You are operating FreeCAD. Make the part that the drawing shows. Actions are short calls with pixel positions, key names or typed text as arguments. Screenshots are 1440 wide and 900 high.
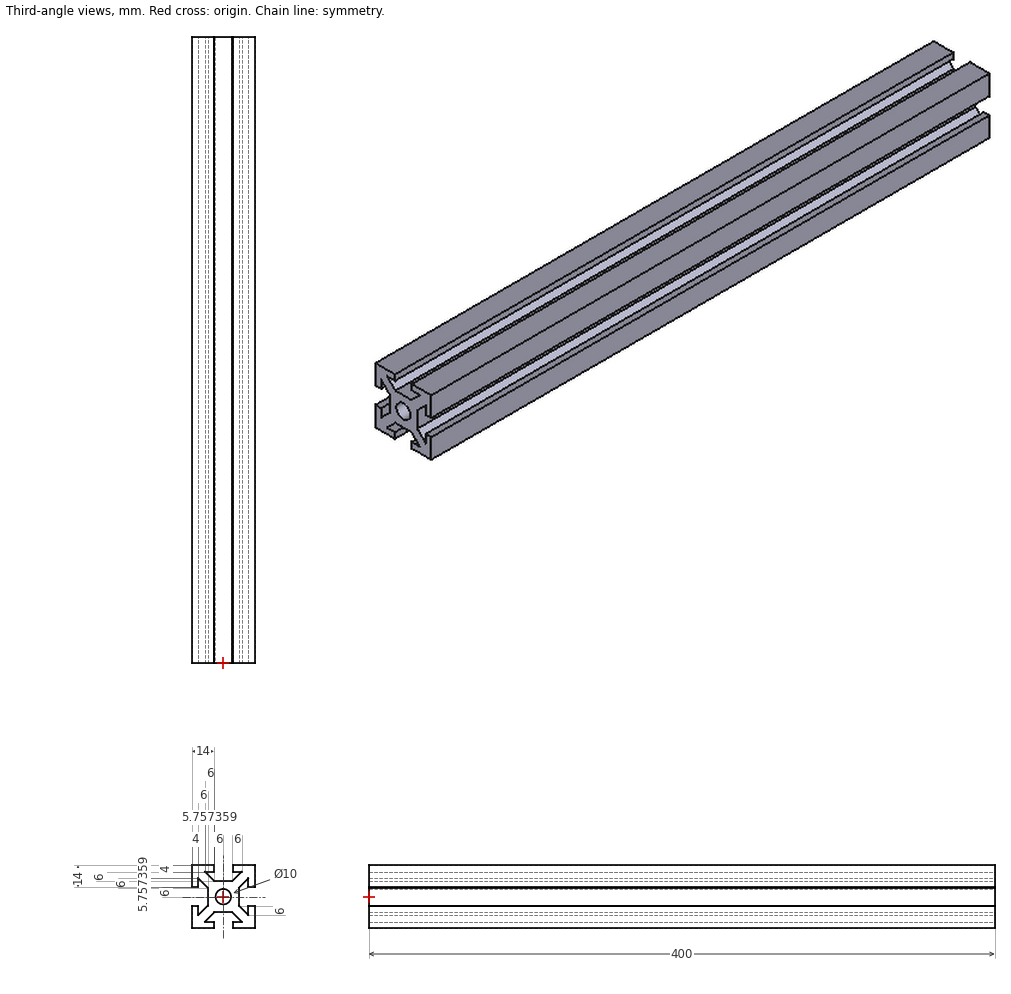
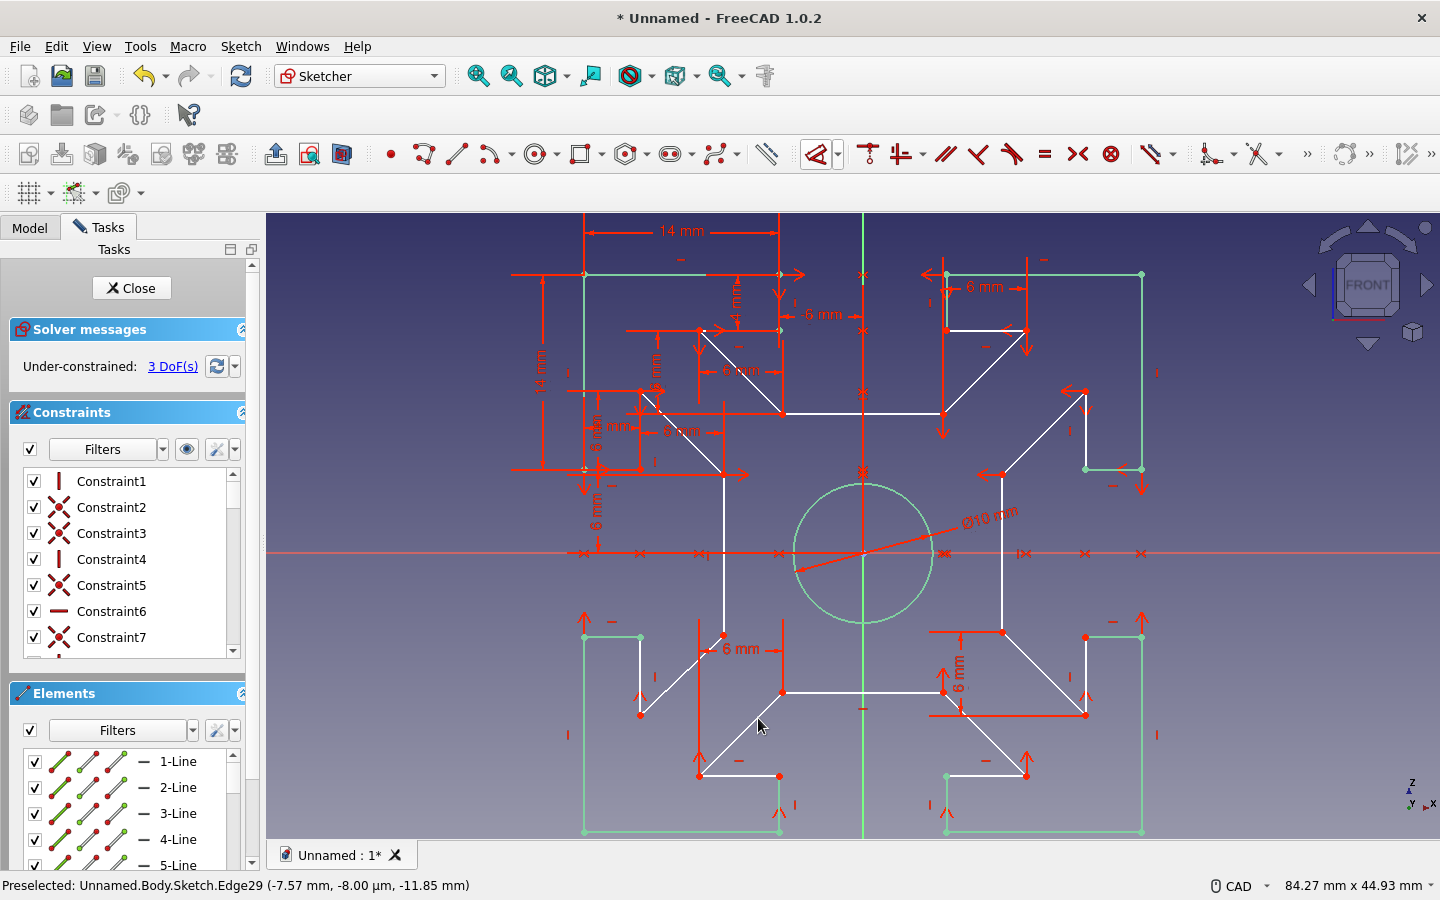
click(665, 692)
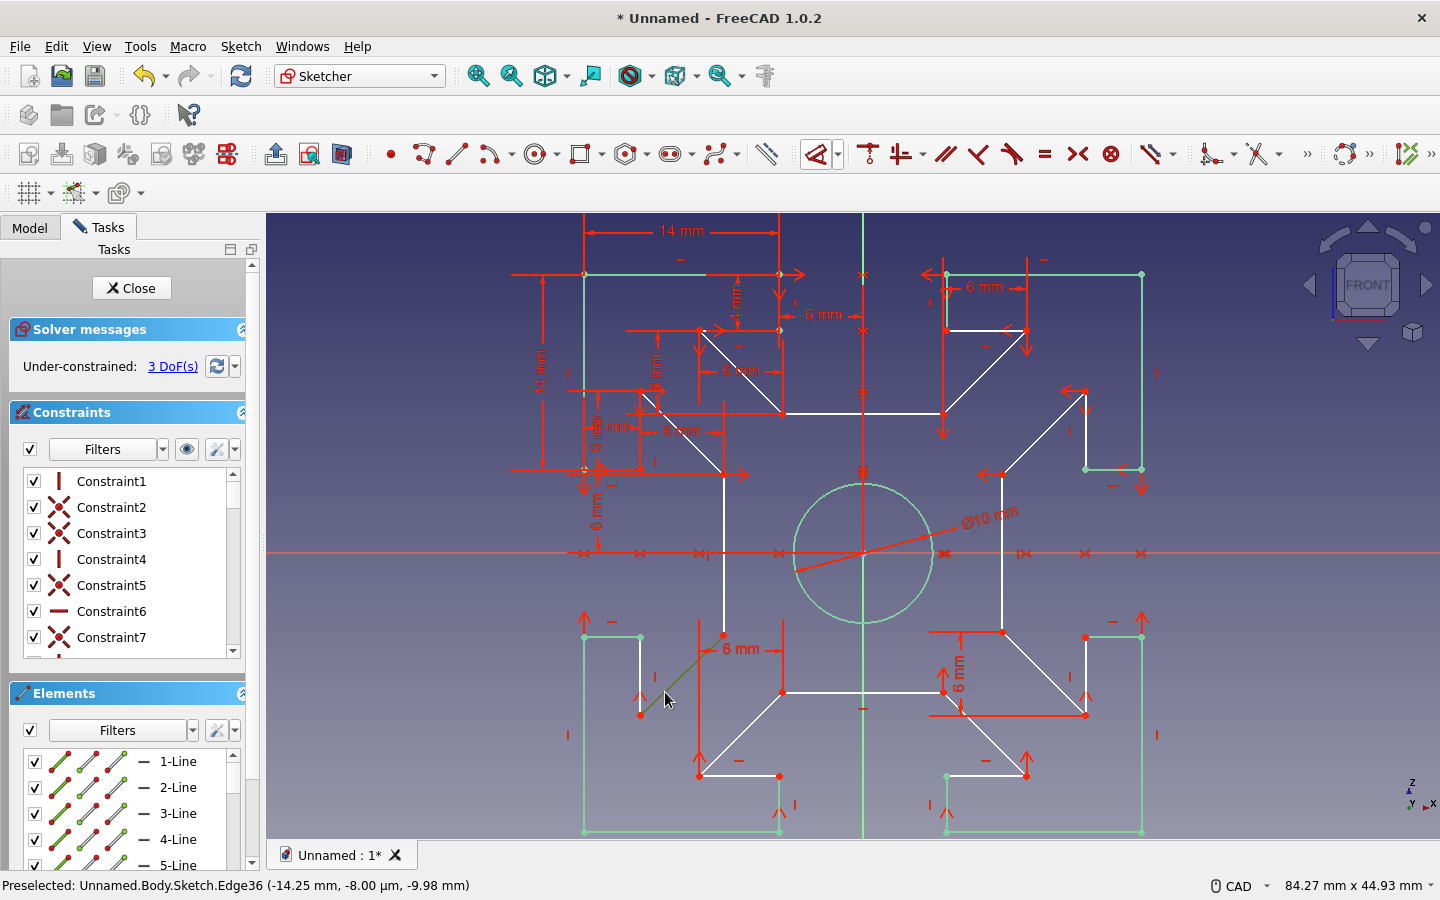
click(838, 154)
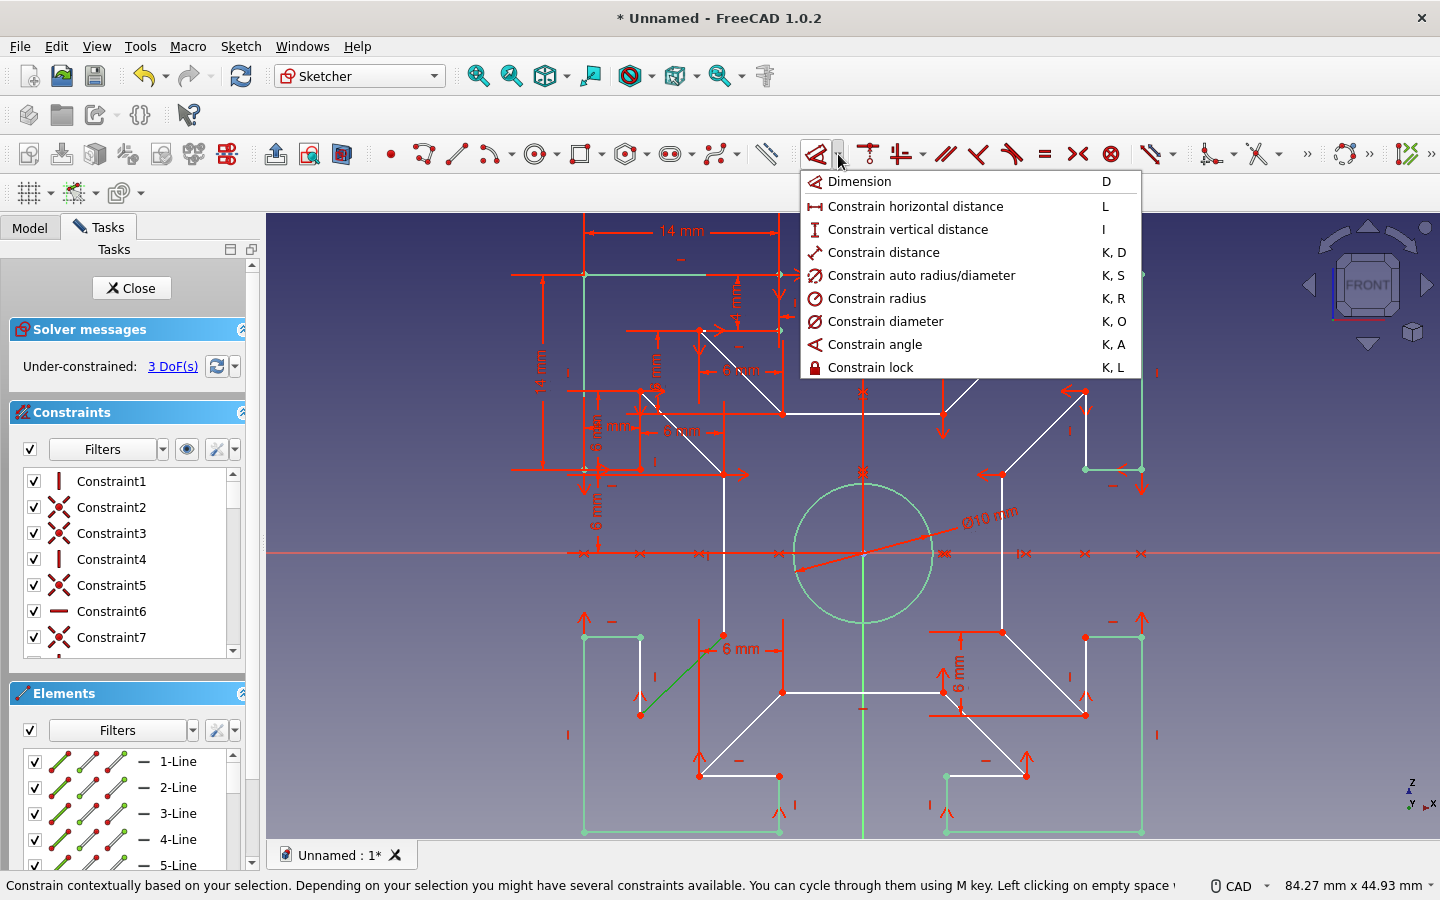
click(971, 230)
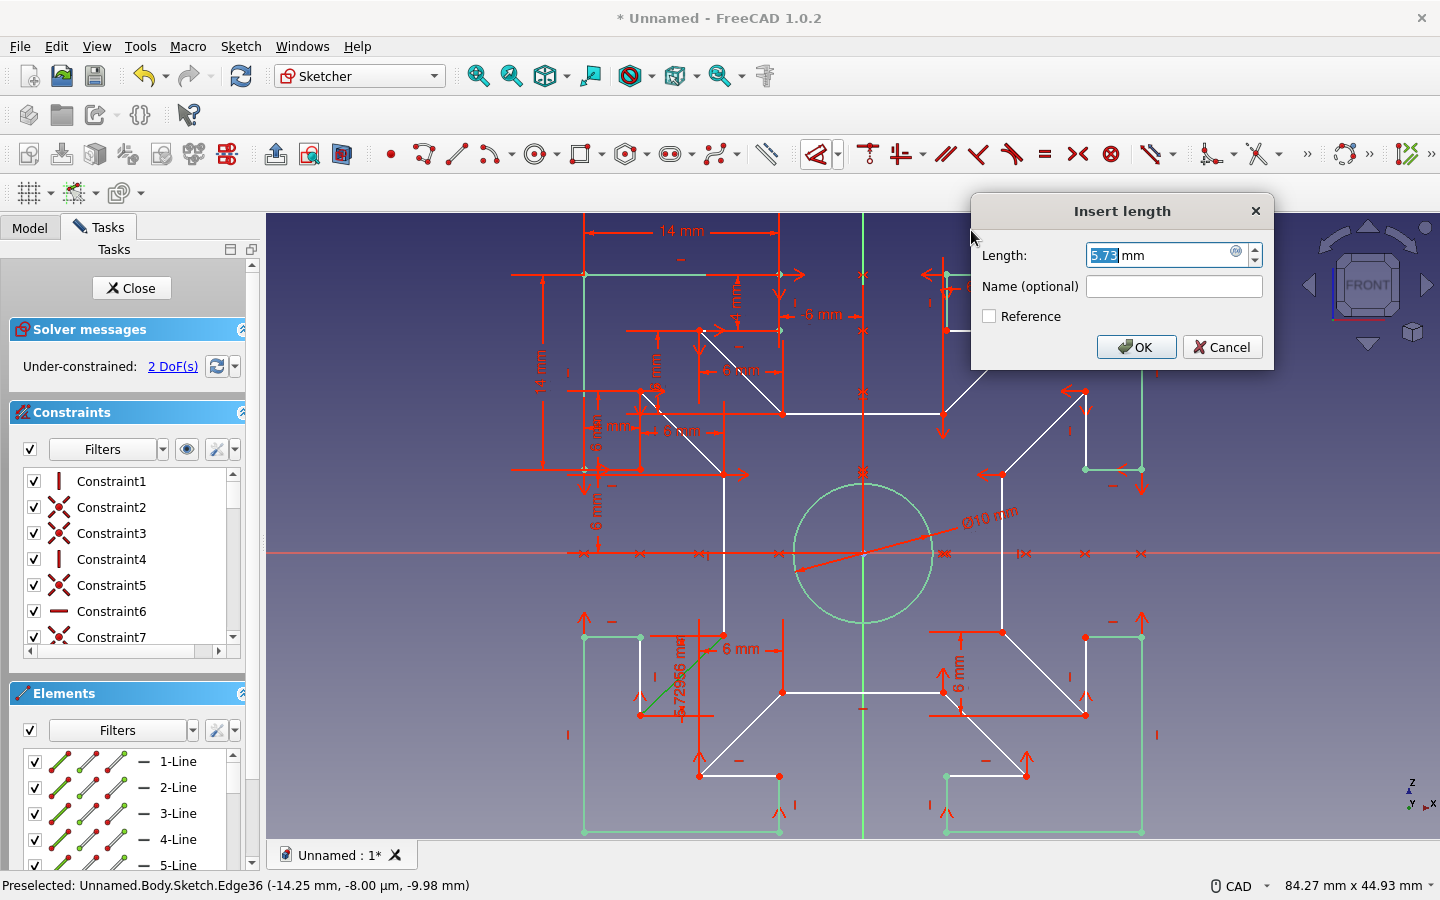
text(6)
key(Return)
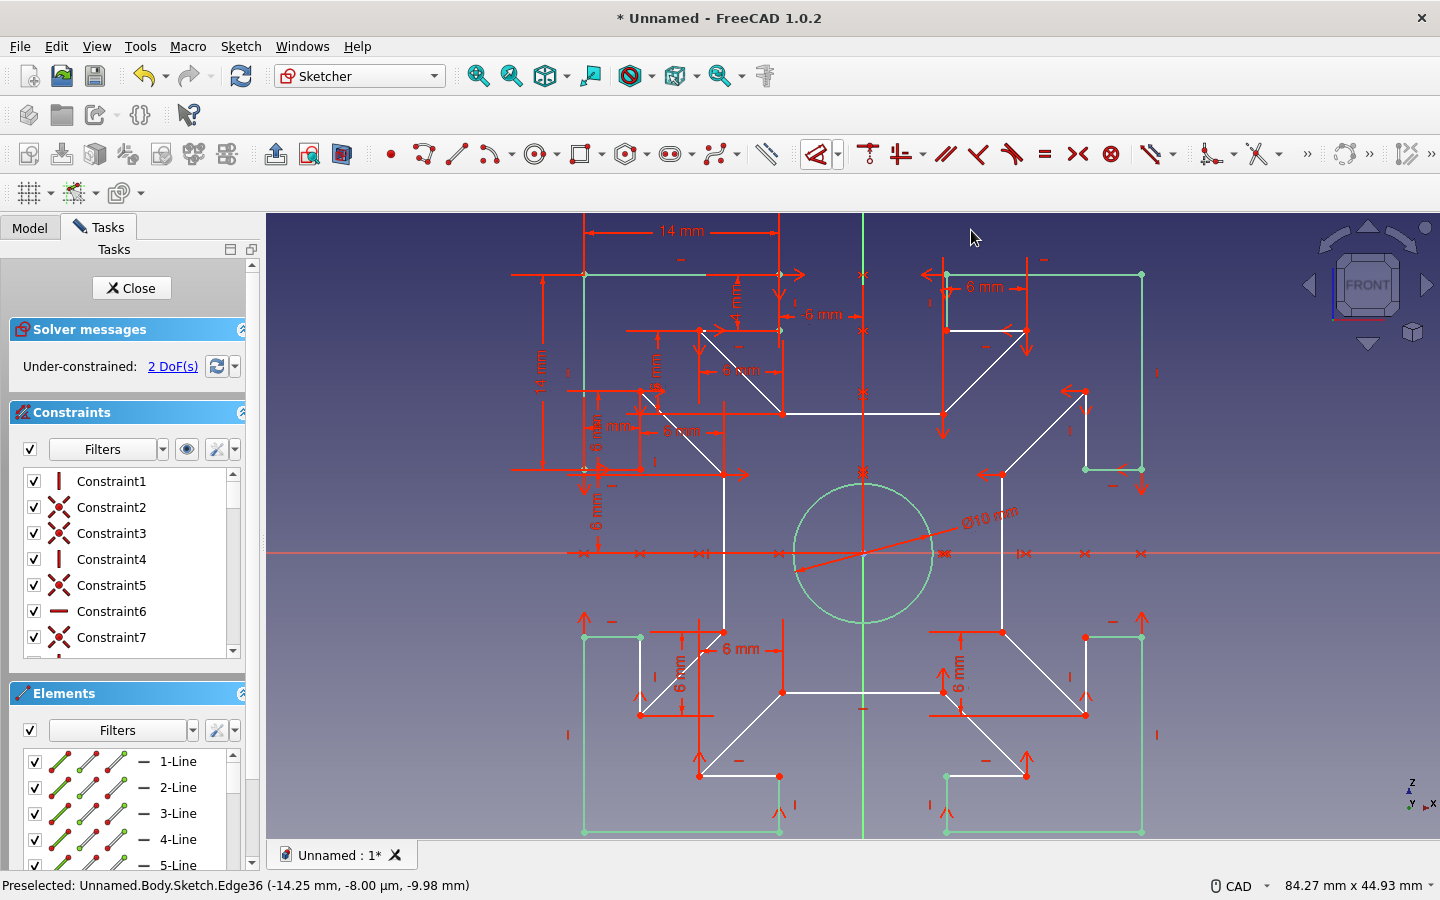
click(640, 446)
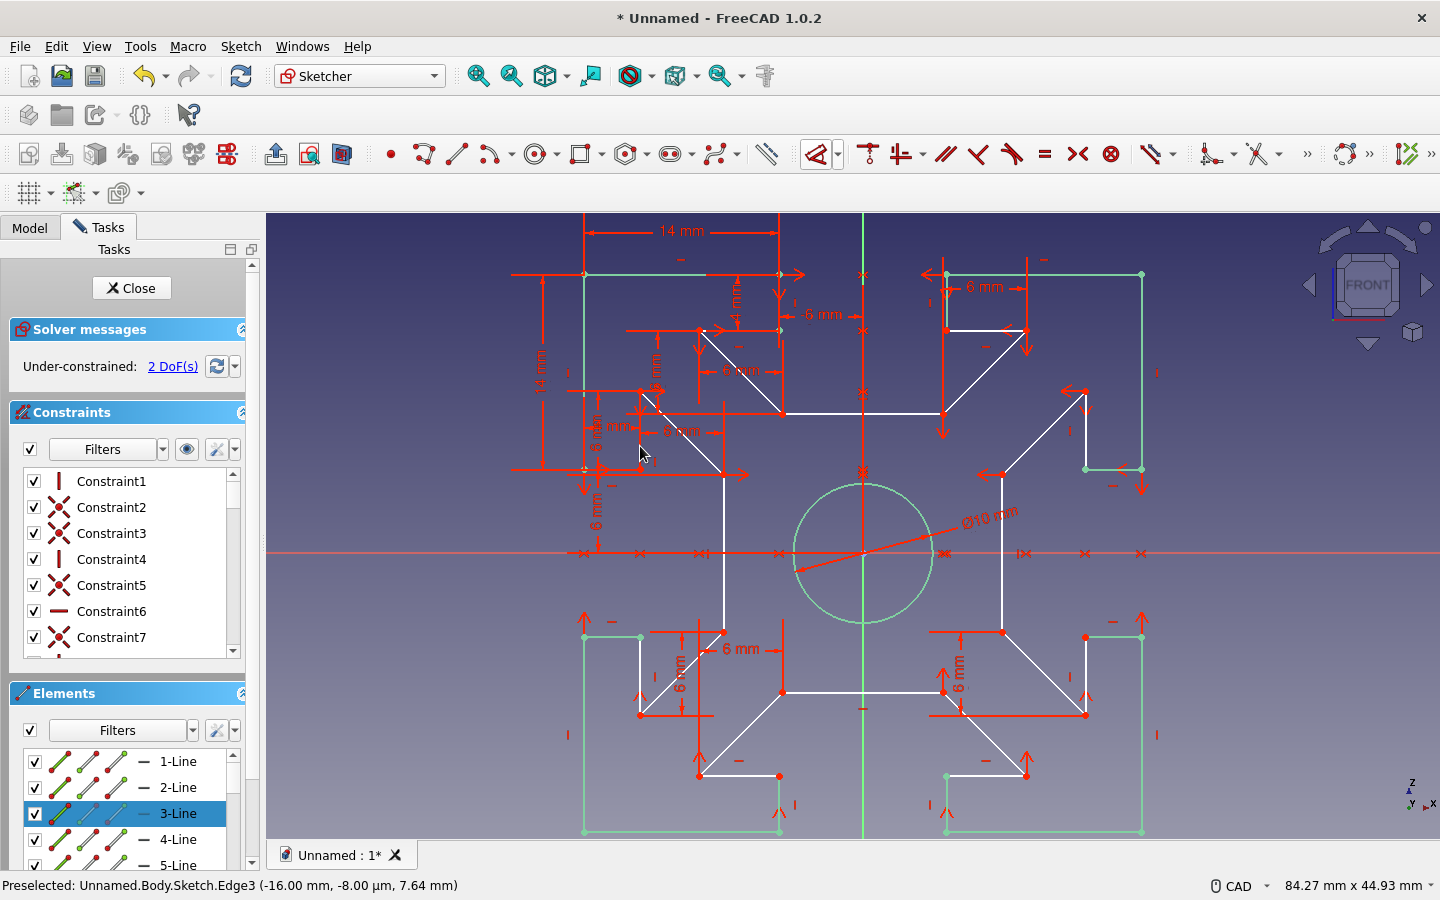
key(i)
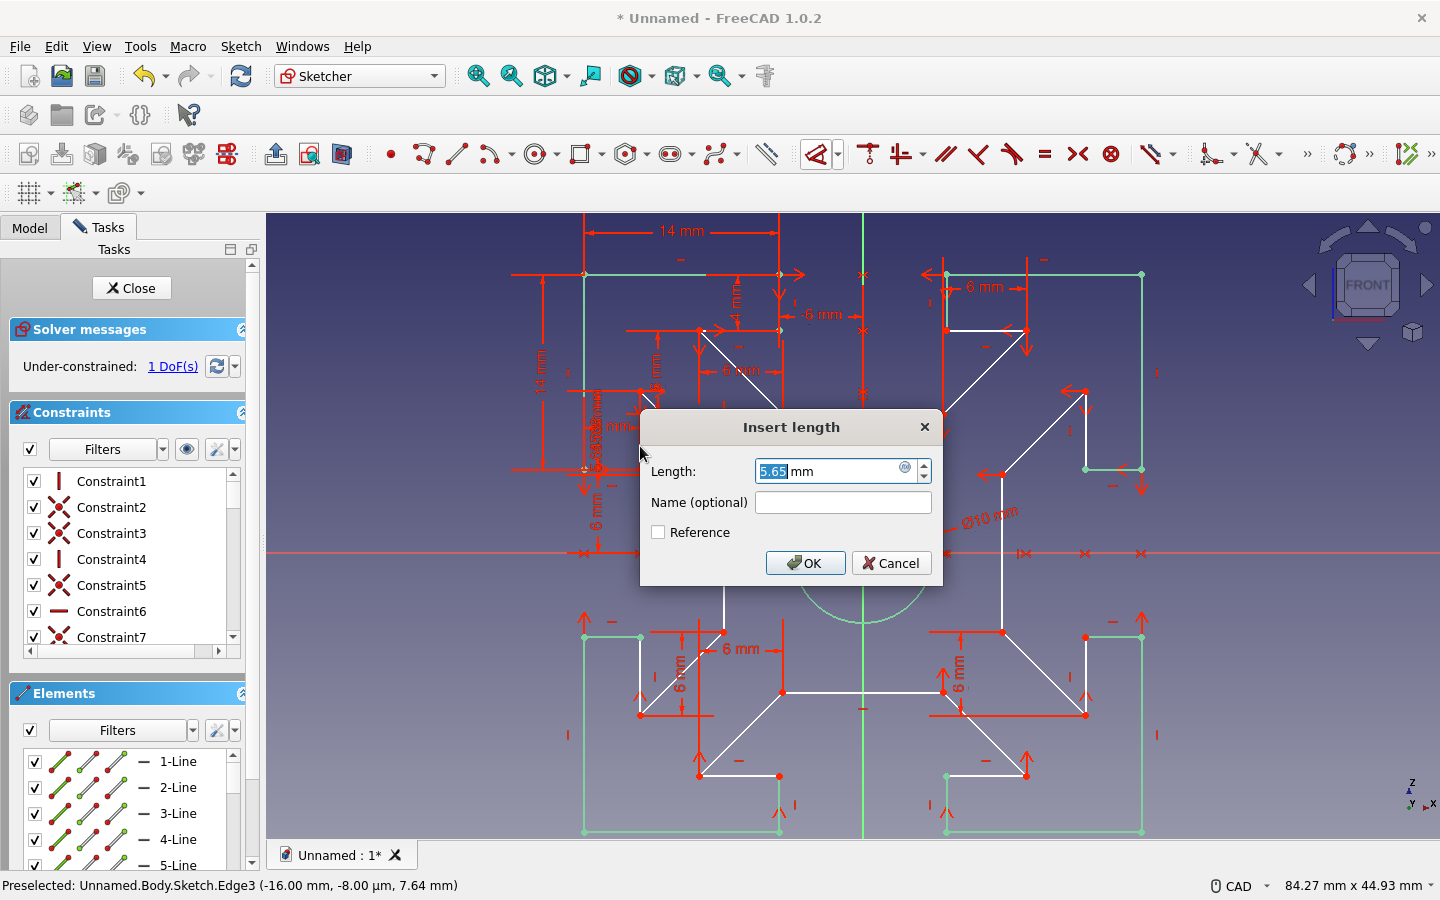
text(5.757359)
key(Return)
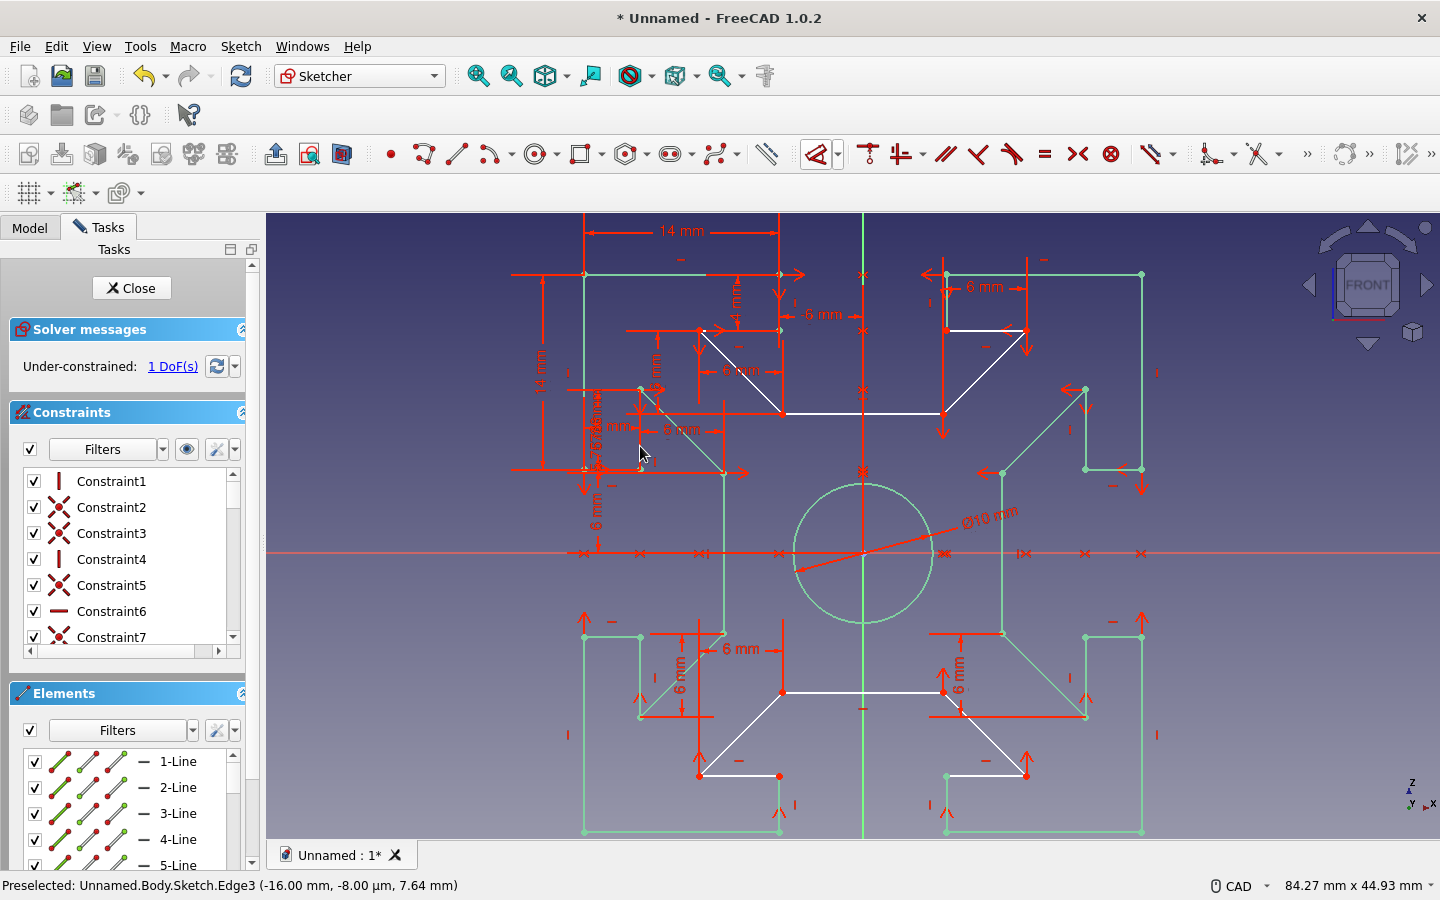
click(755, 331)